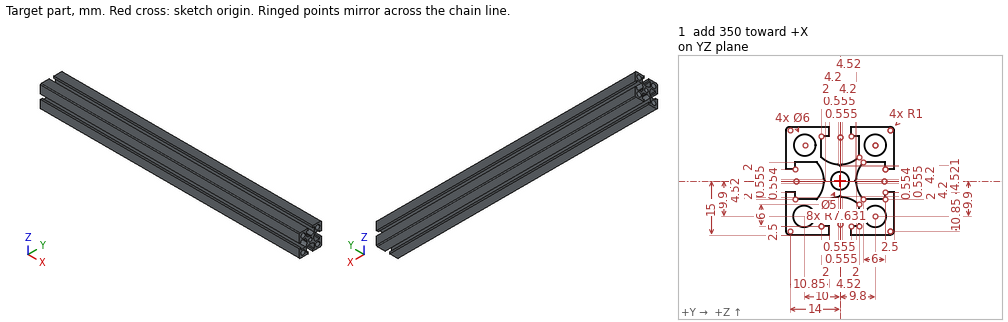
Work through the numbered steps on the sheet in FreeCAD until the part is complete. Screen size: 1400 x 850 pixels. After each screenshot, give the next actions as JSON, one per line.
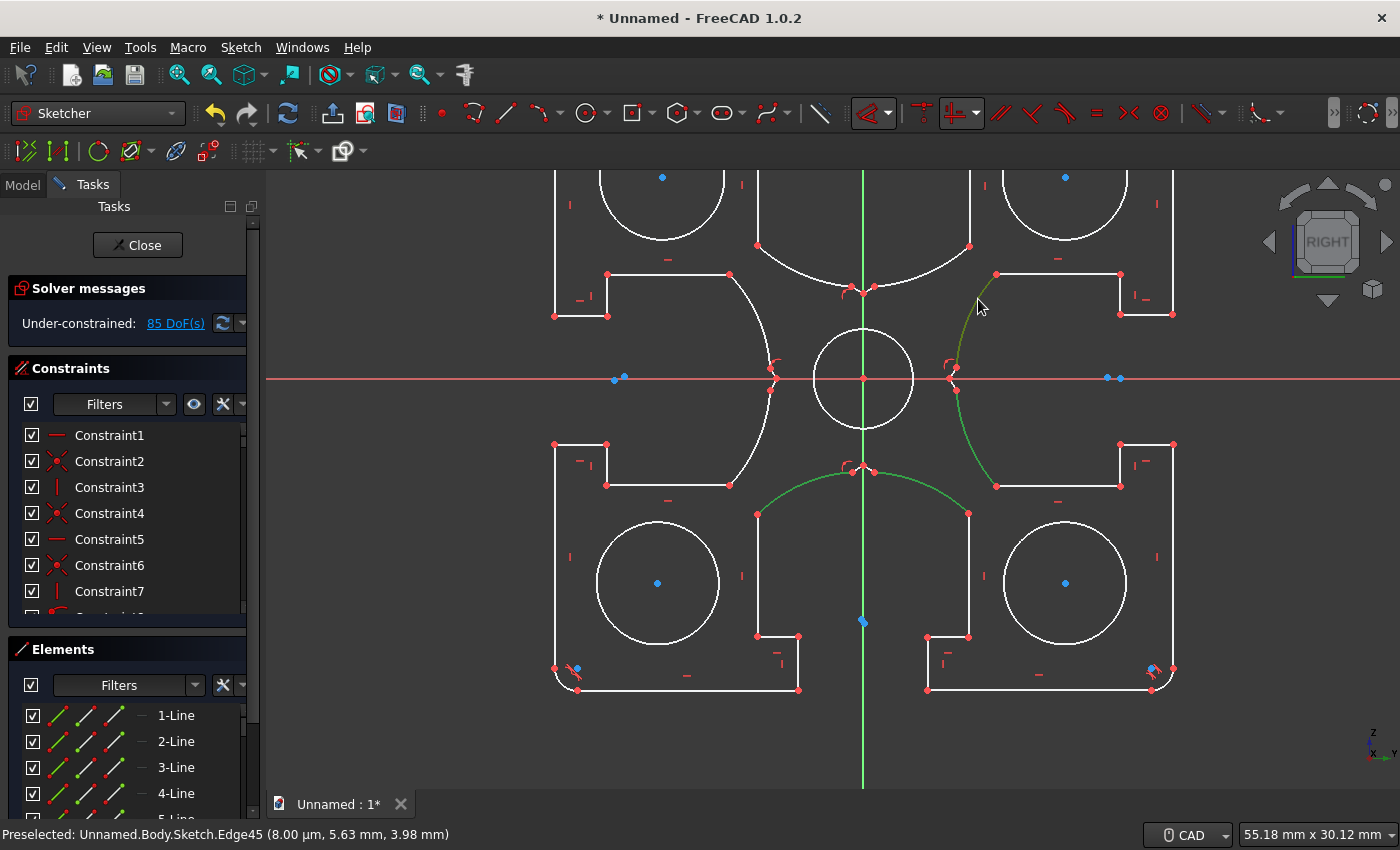
{"action": "left_click", "coordinate": [905, 281]}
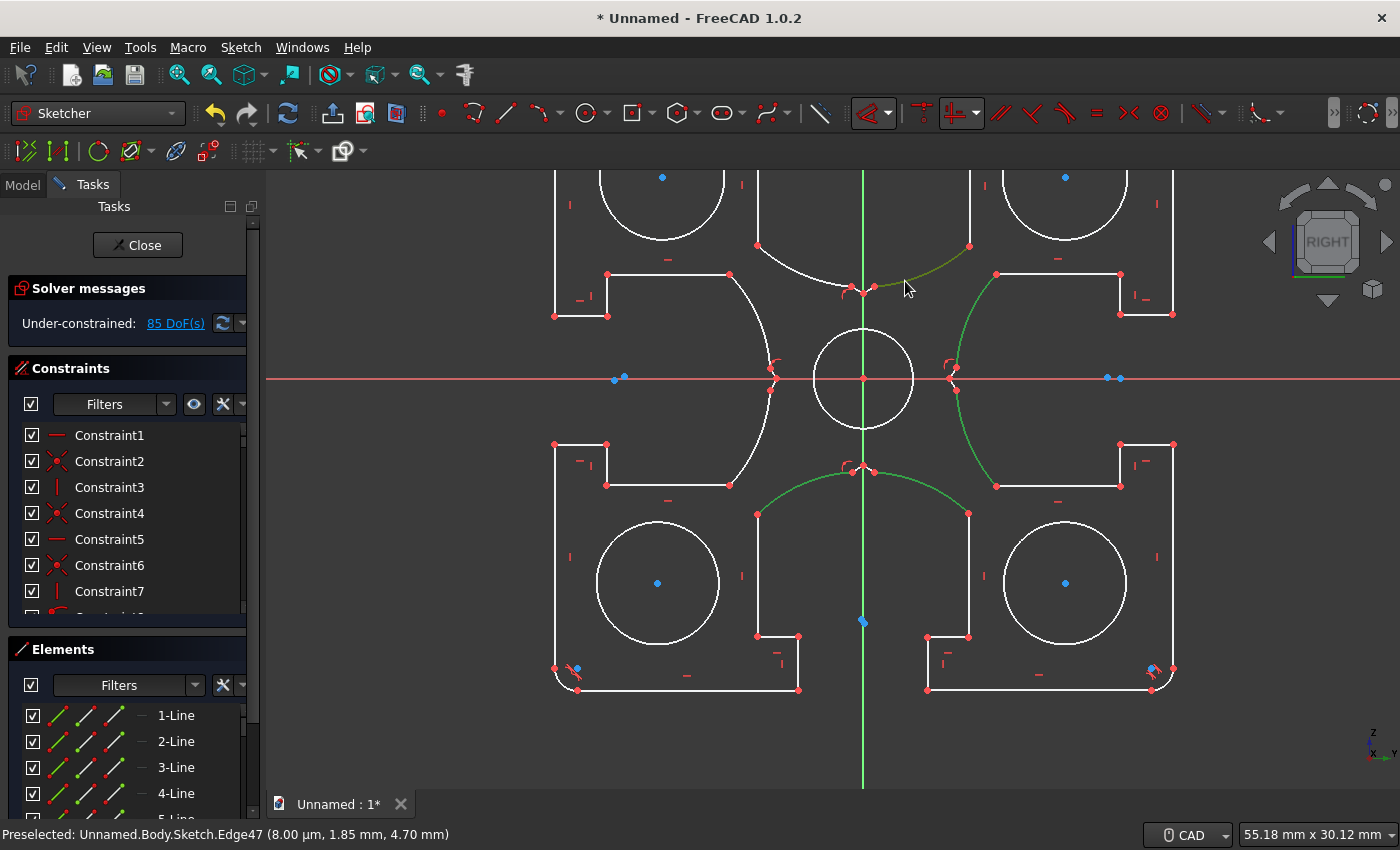
{"action": "left_click", "coordinate": [783, 264]}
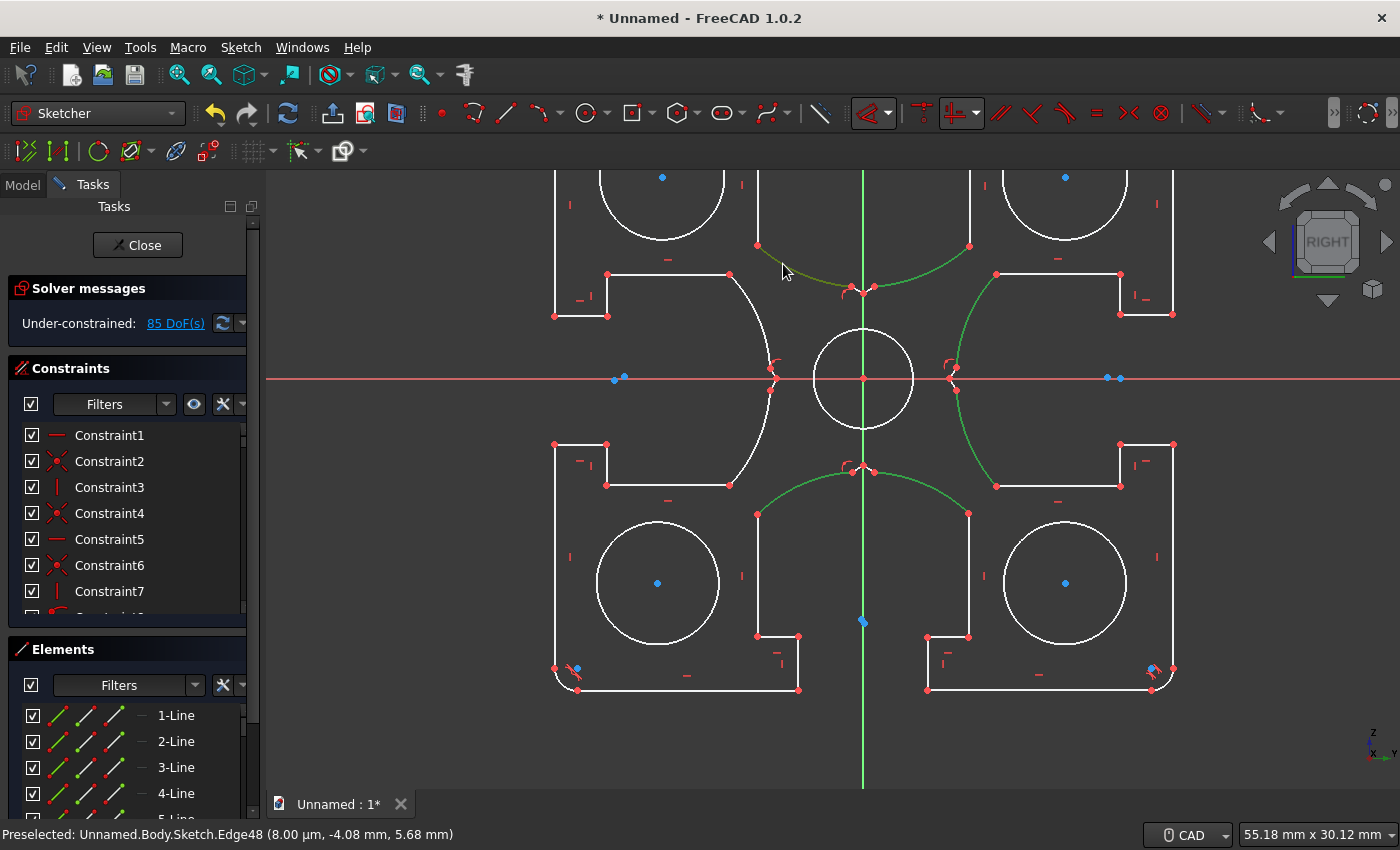
{"action": "left_click", "coordinate": [765, 337]}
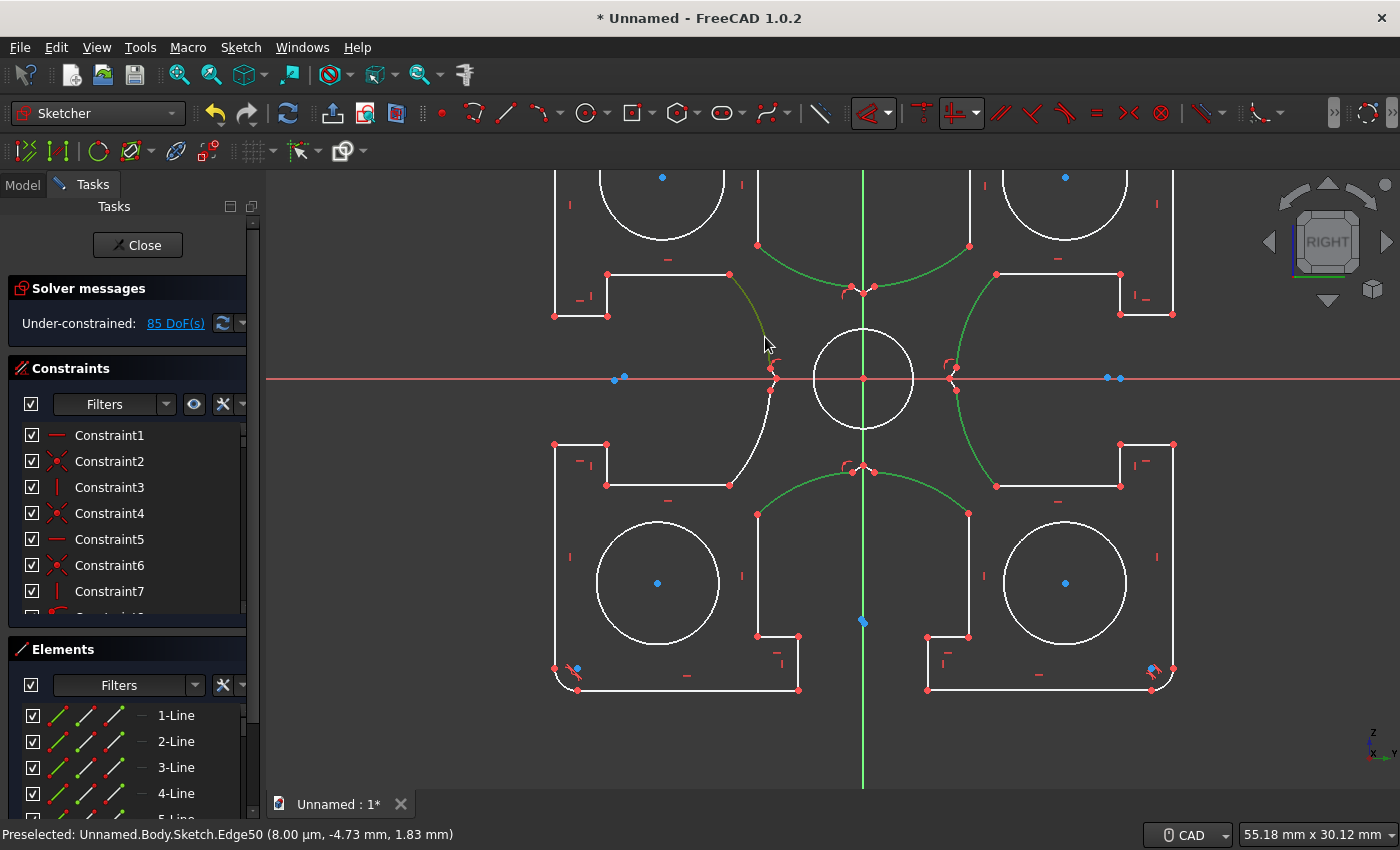
{"action": "left_click", "coordinate": [749, 460]}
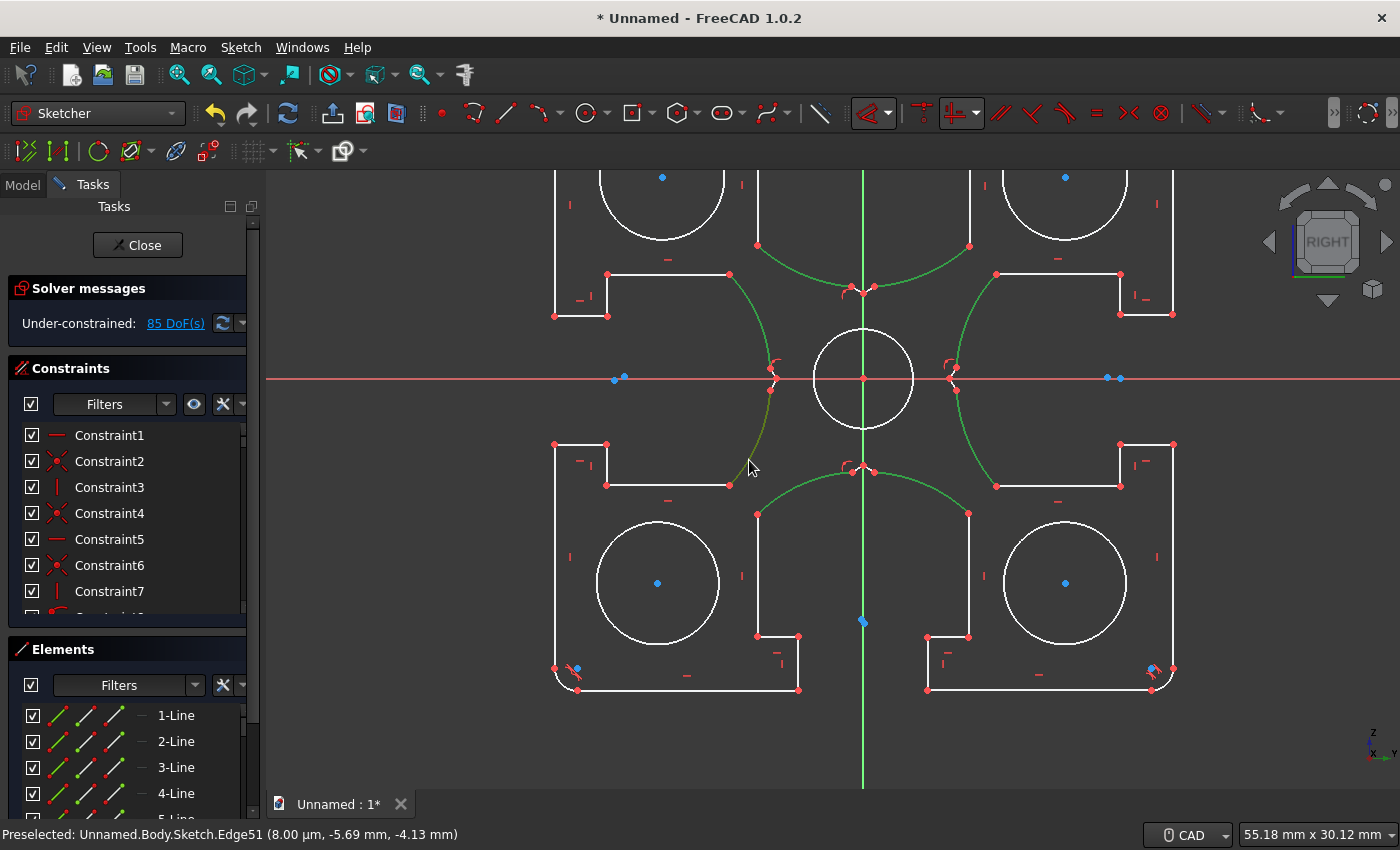
{"action": "key", "text": "e"}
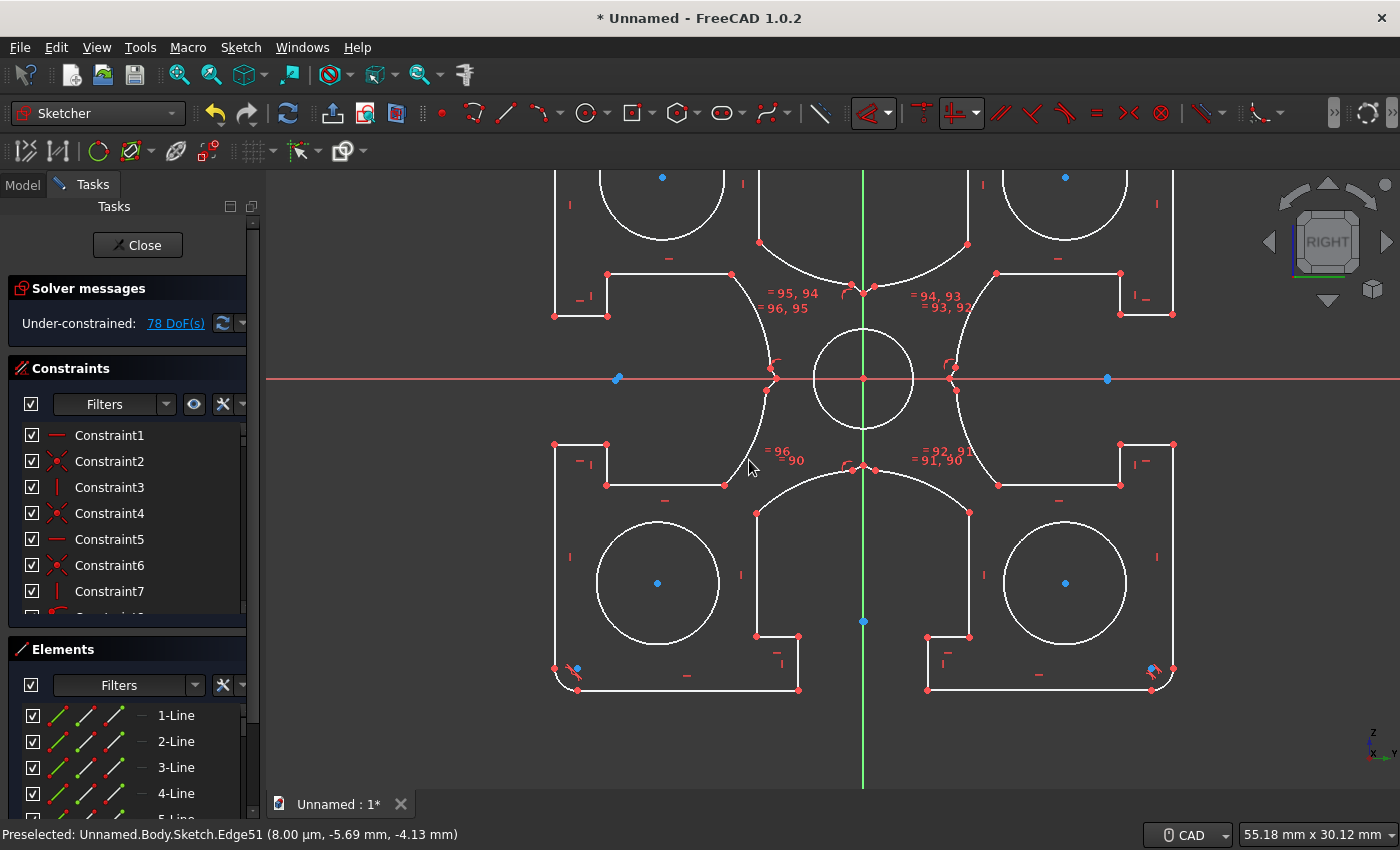
{"action": "scroll", "coordinate": [1161, 688], "scroll_direction": "up", "scroll_amount": 2}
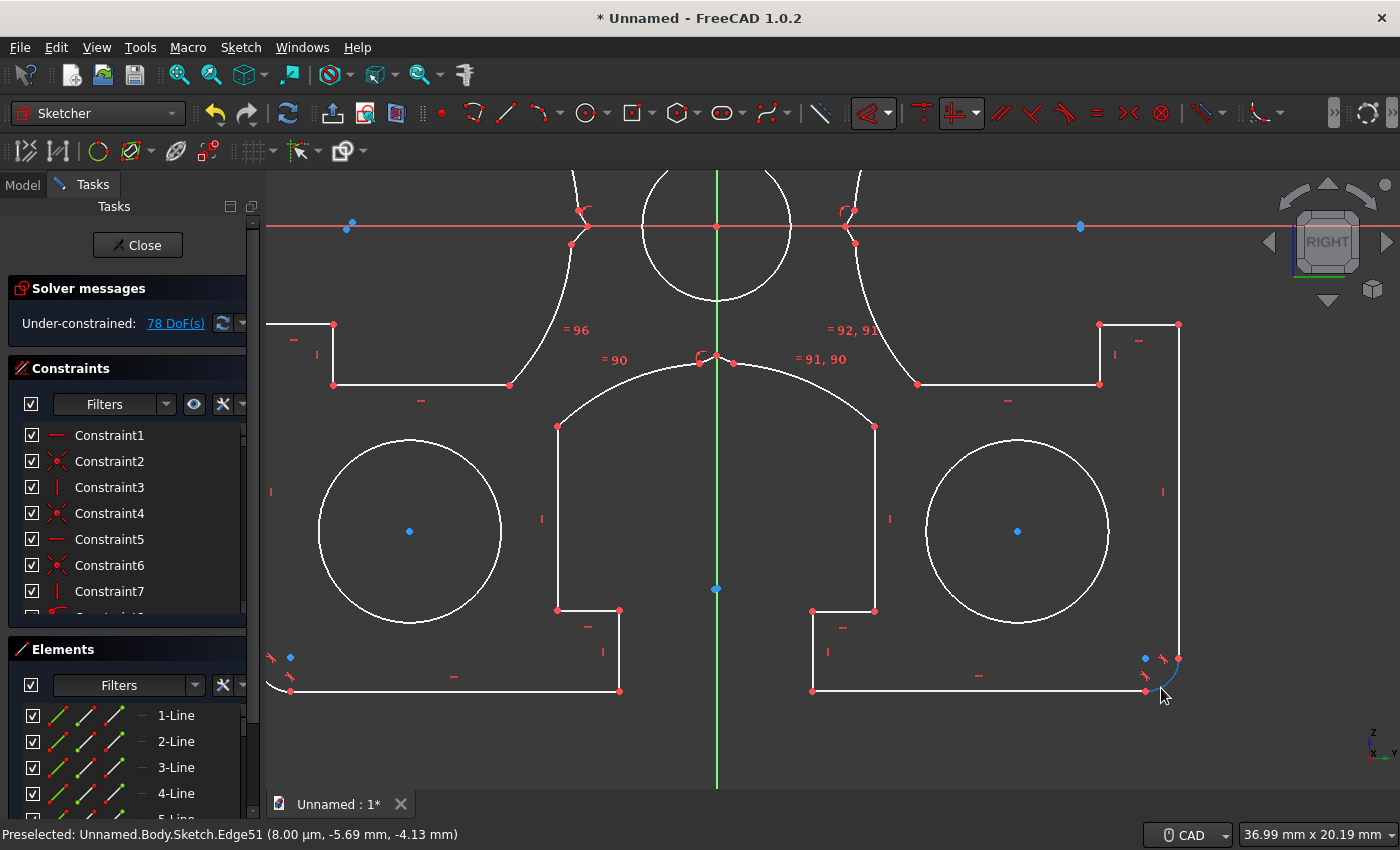
{"action": "left_click", "coordinate": [1161, 688]}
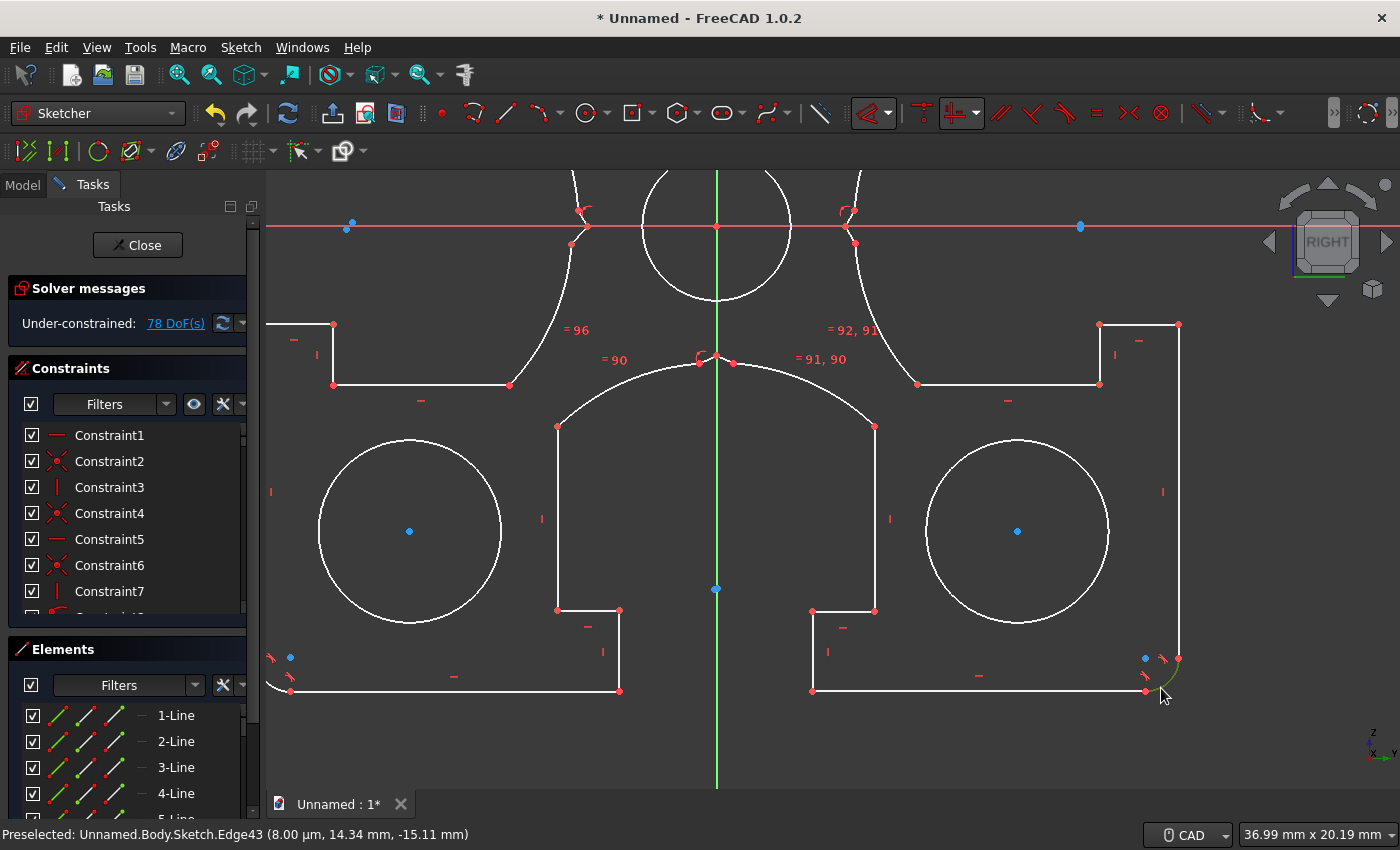
{"action": "scroll", "coordinate": [804, 686], "scroll_direction": "down", "scroll_amount": 4}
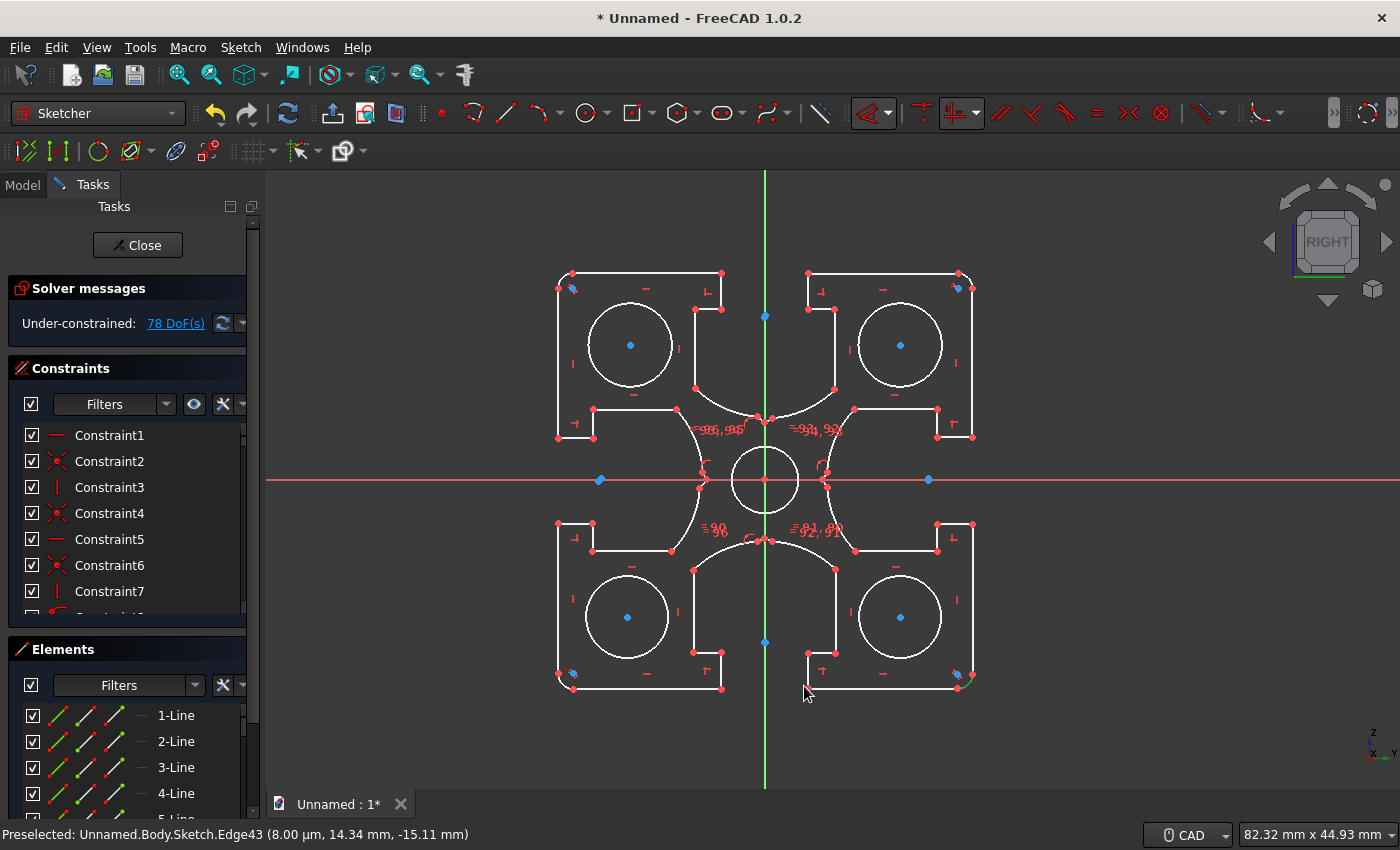
{"action": "scroll", "coordinate": [971, 282], "scroll_direction": "up", "scroll_amount": 4}